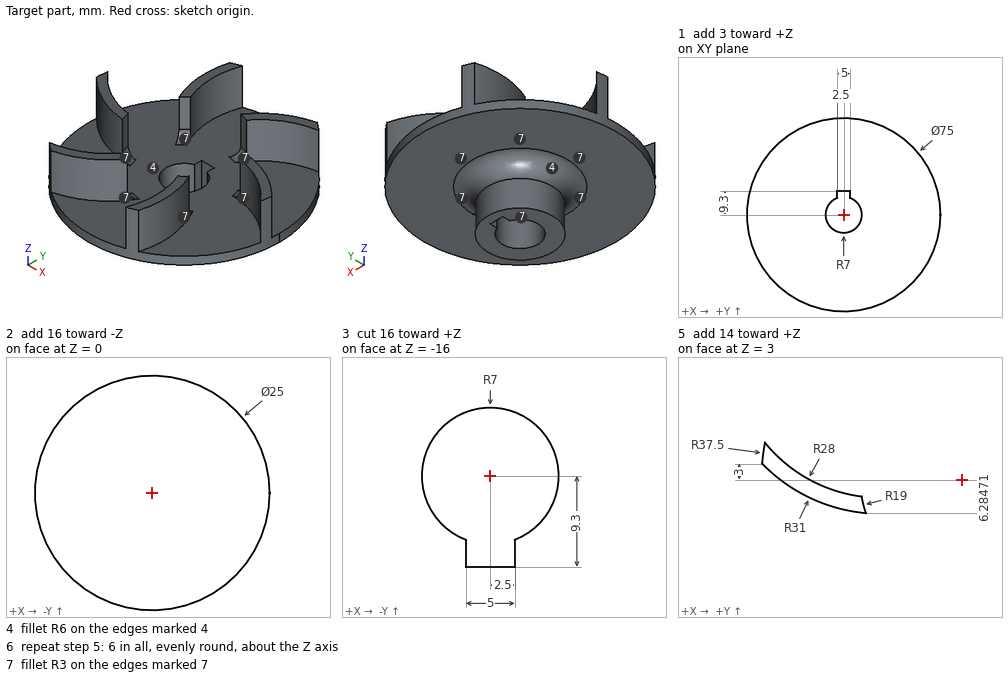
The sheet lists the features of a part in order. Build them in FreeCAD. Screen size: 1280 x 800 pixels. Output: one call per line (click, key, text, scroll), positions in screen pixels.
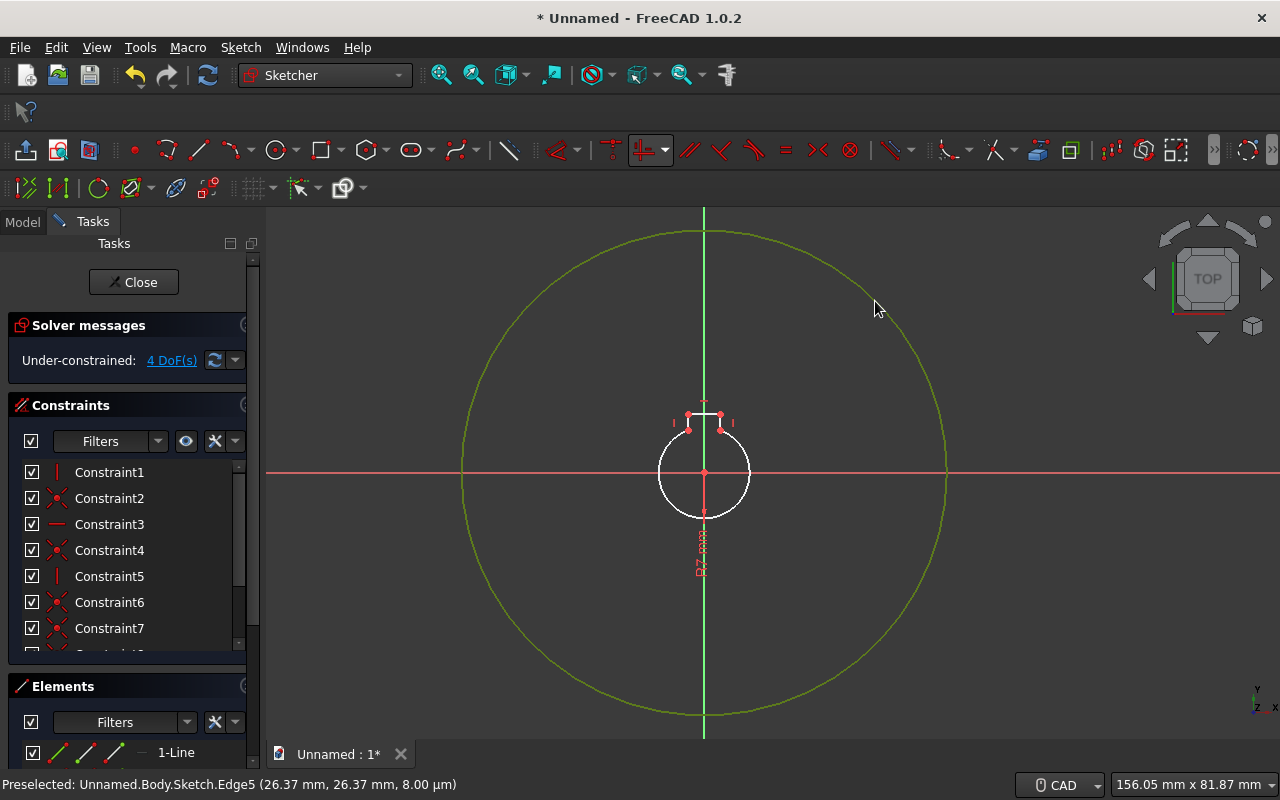
key(k)
key(o)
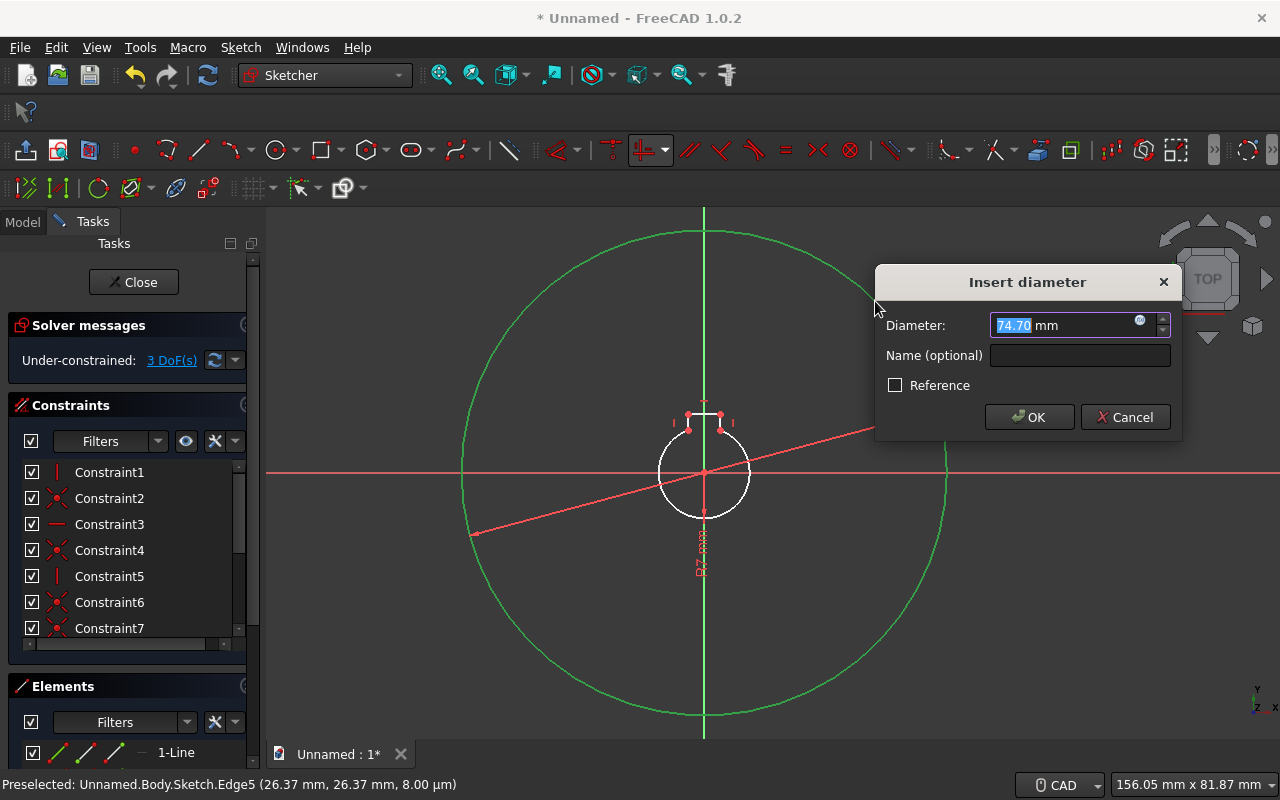
text(75)
key(Return)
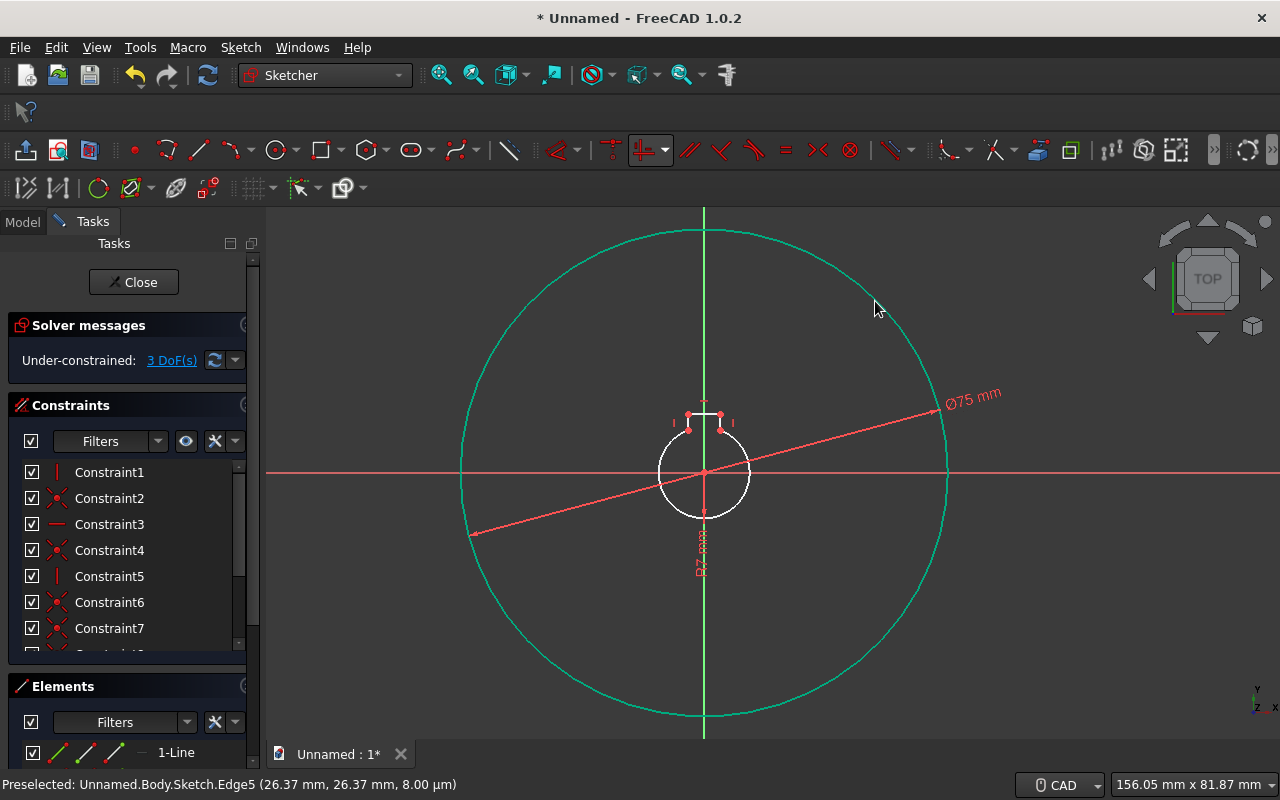
scroll(701, 414, up, 2)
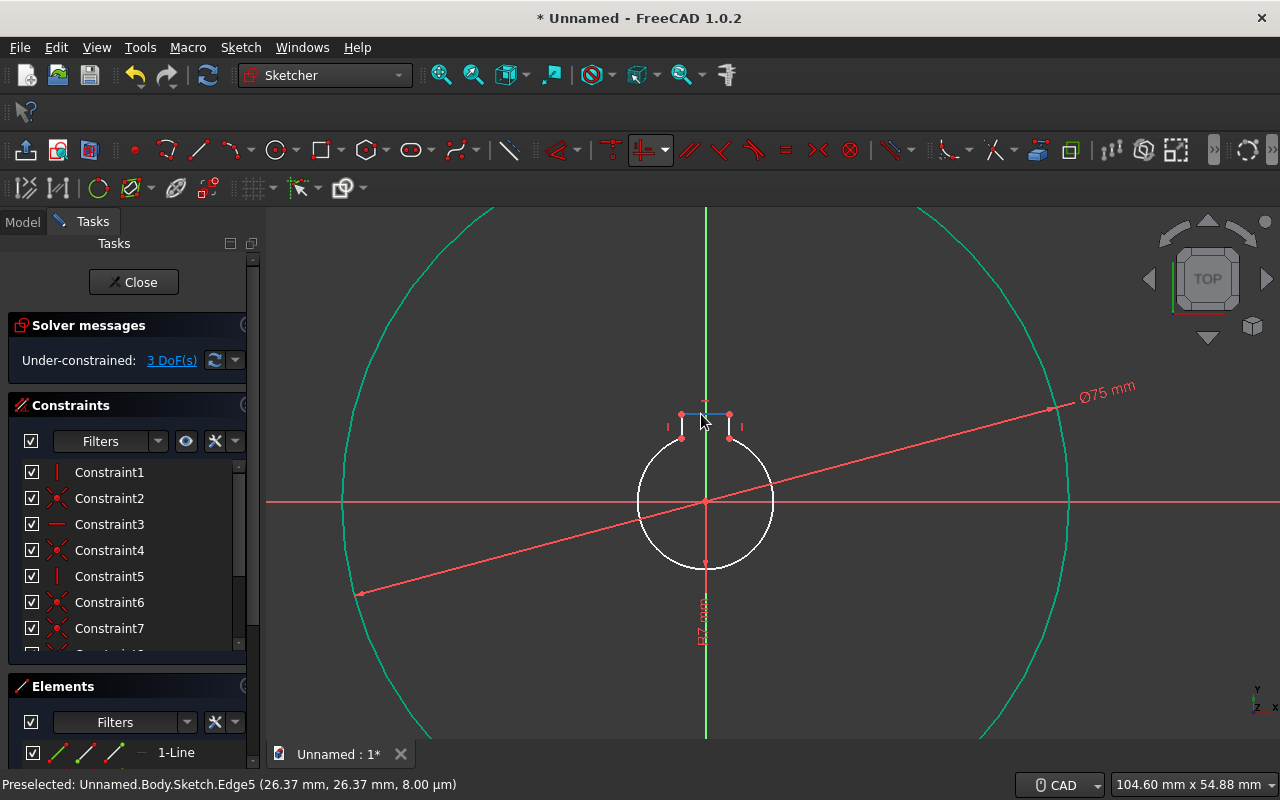
click(701, 414)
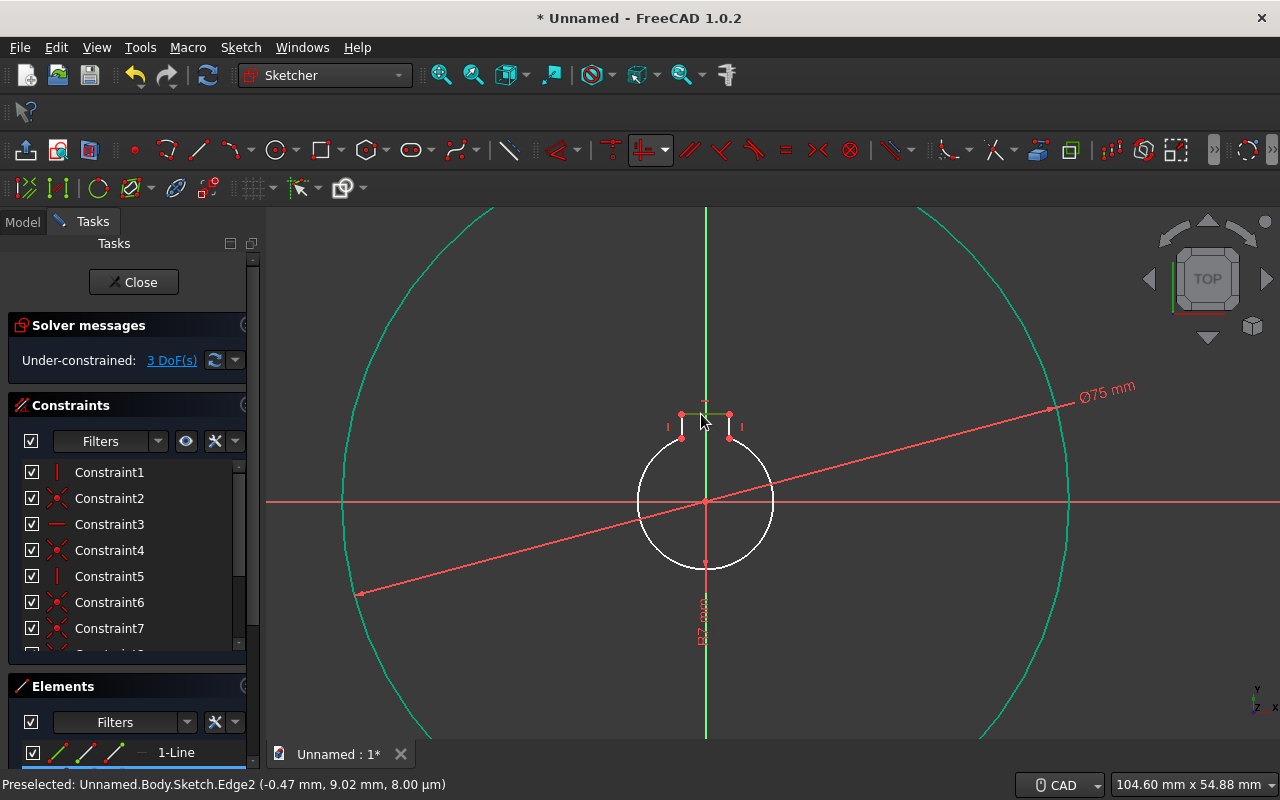
key(l)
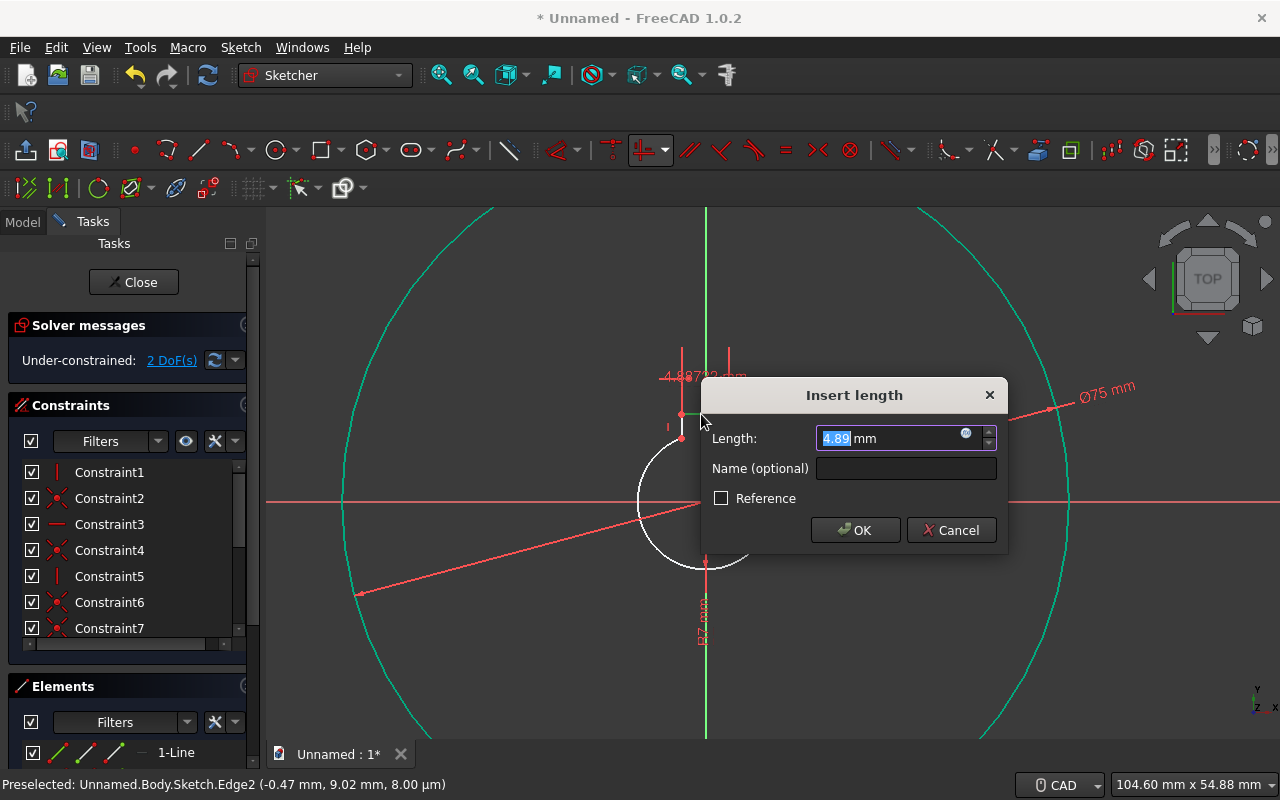
text(5)
key(Return)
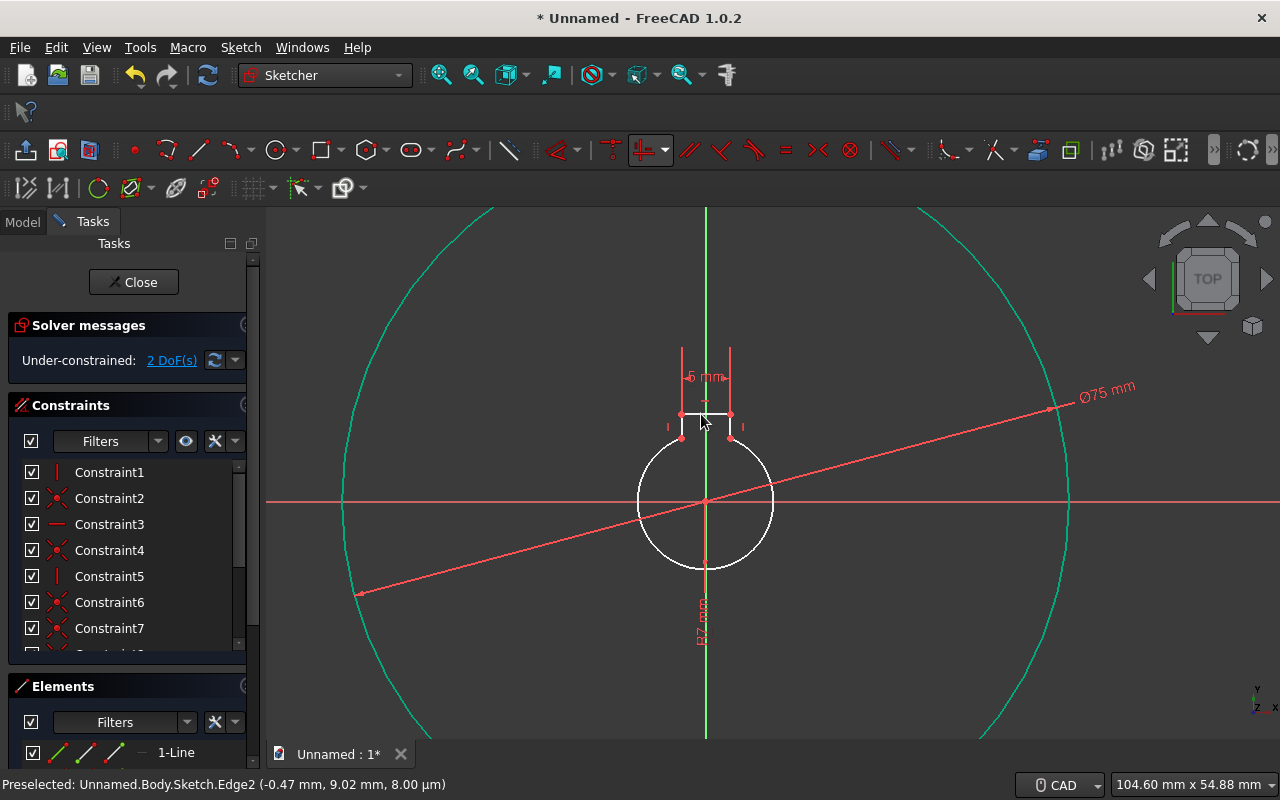
scroll(682, 438, up, 3)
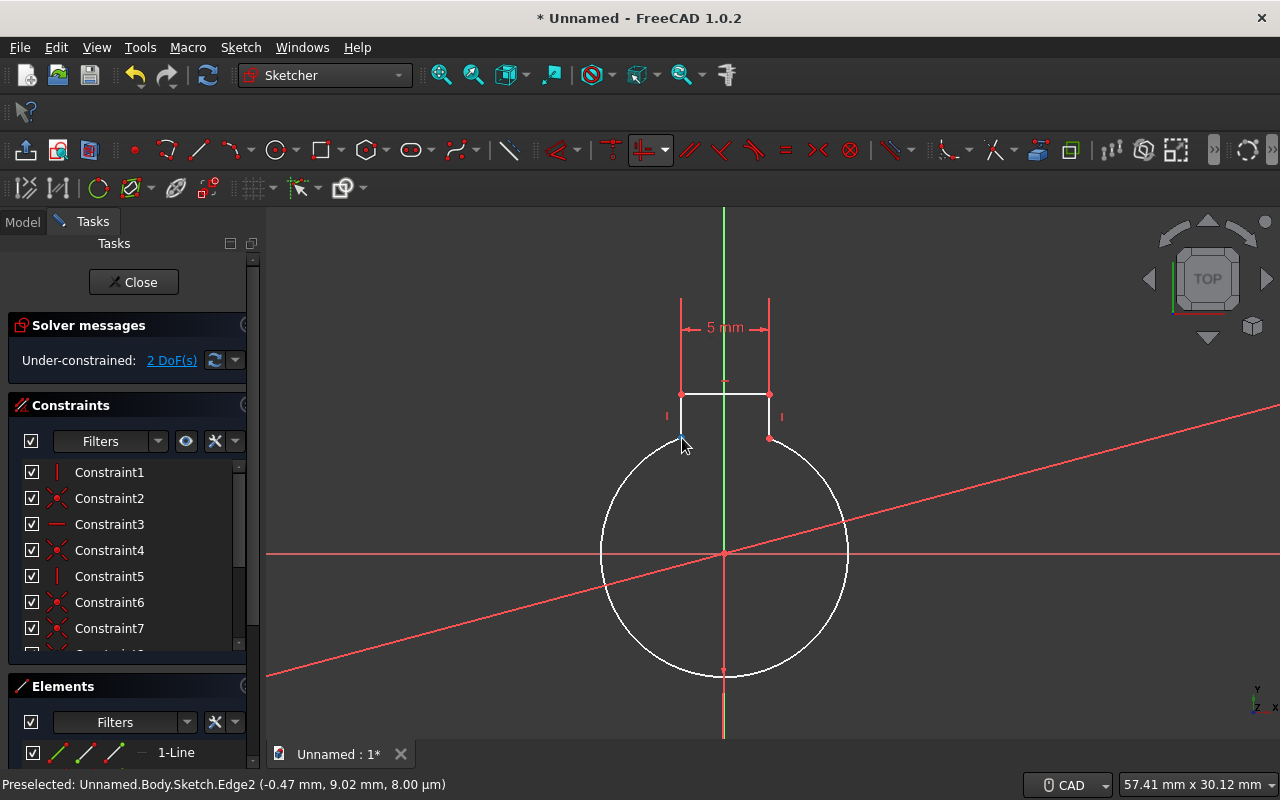
click(681, 438)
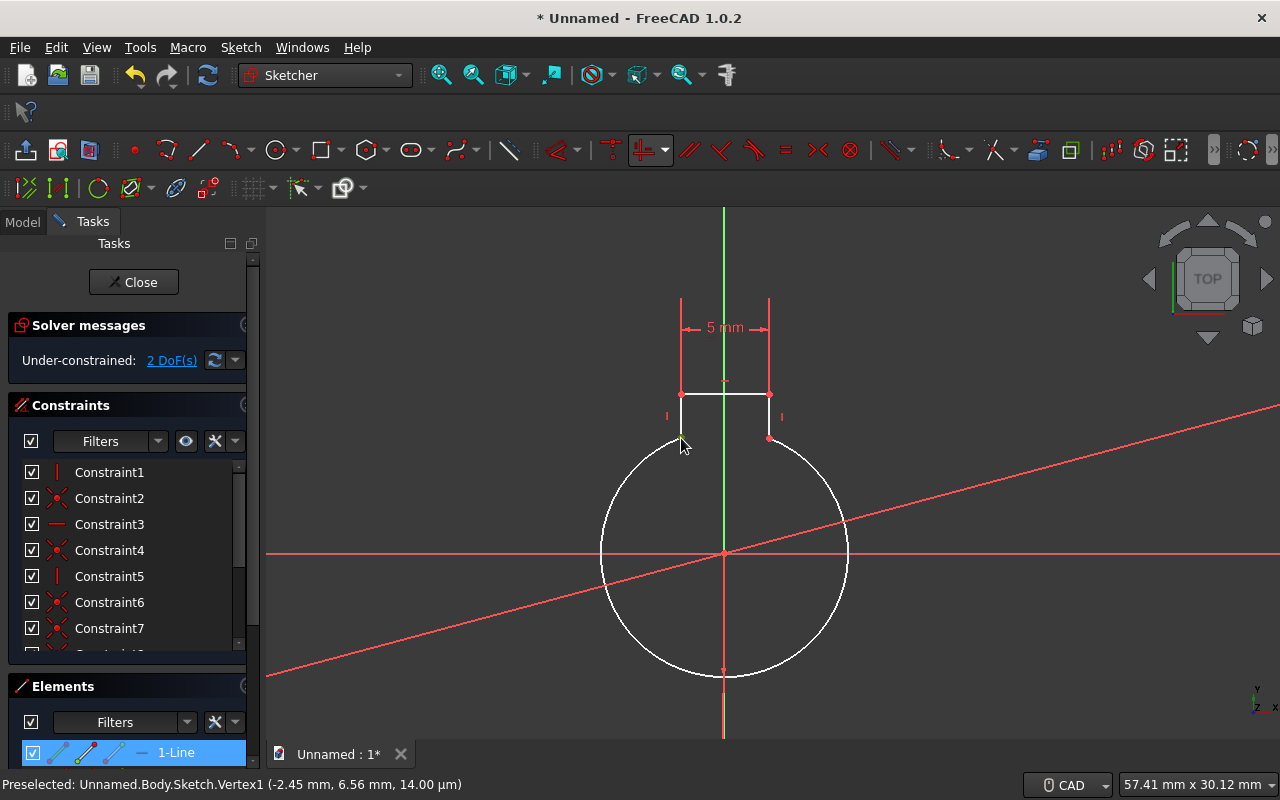
key(l)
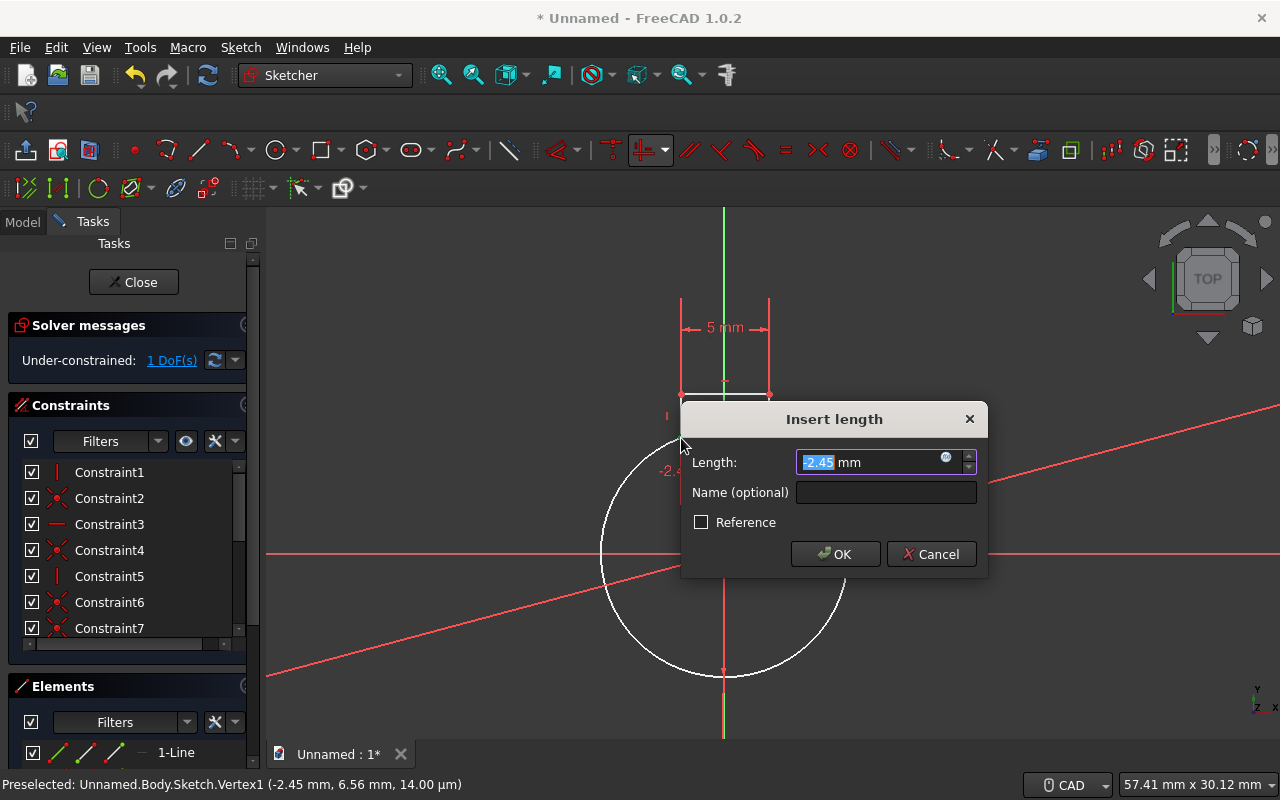
text(-2.5)
key(Return)